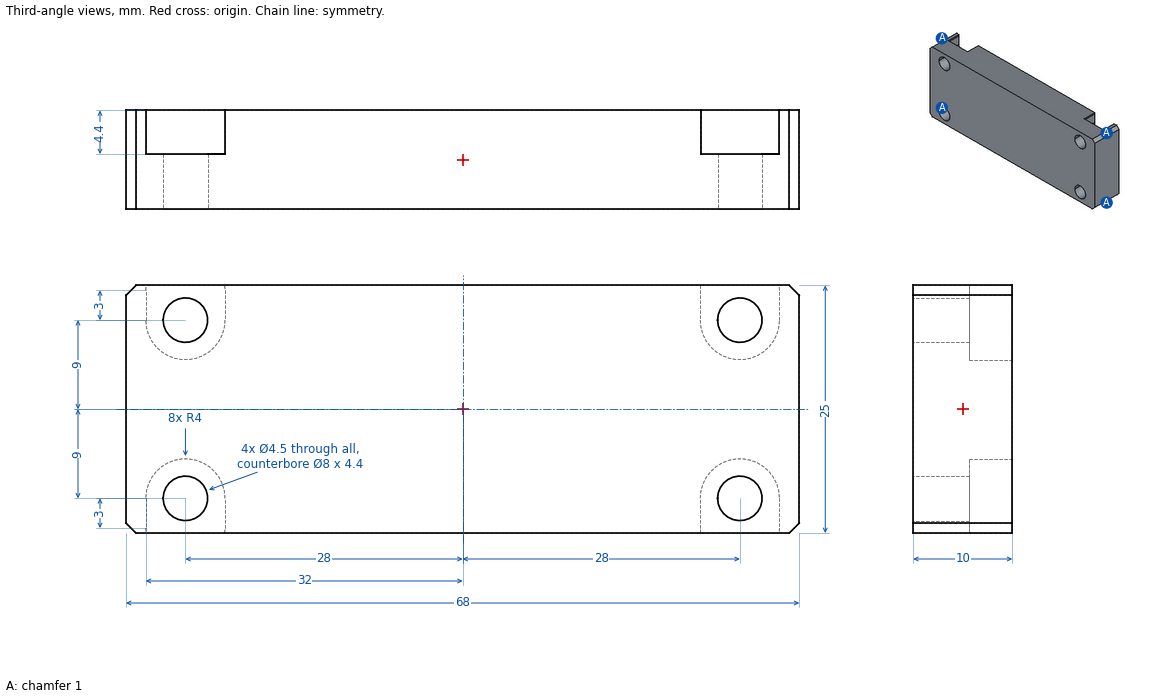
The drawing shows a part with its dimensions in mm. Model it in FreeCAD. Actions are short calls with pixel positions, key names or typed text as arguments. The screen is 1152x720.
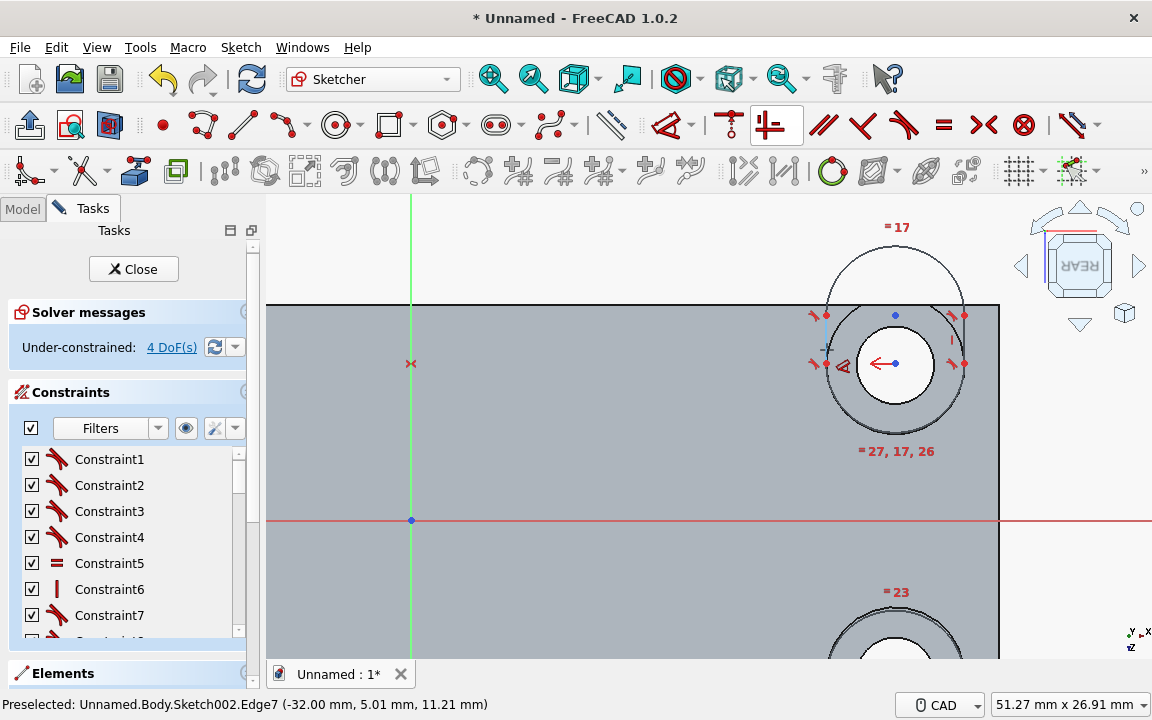
click(826, 349)
click(860, 340)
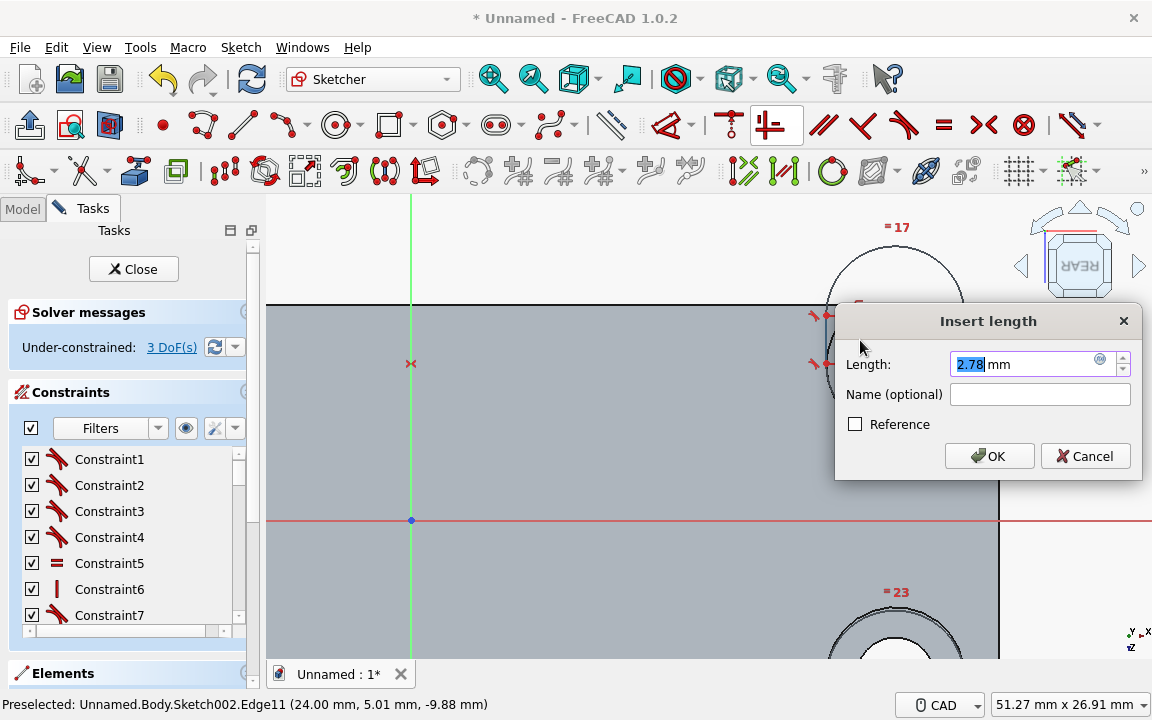
text(3)
key(Return)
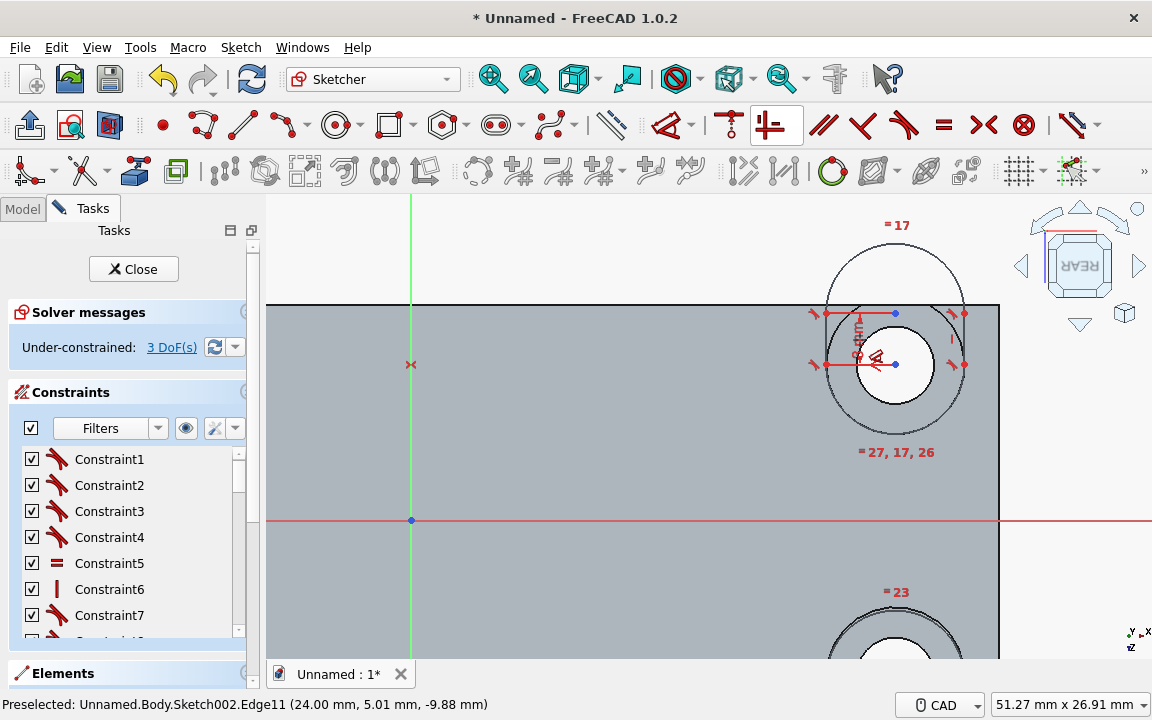
scroll(827, 350, down, 4)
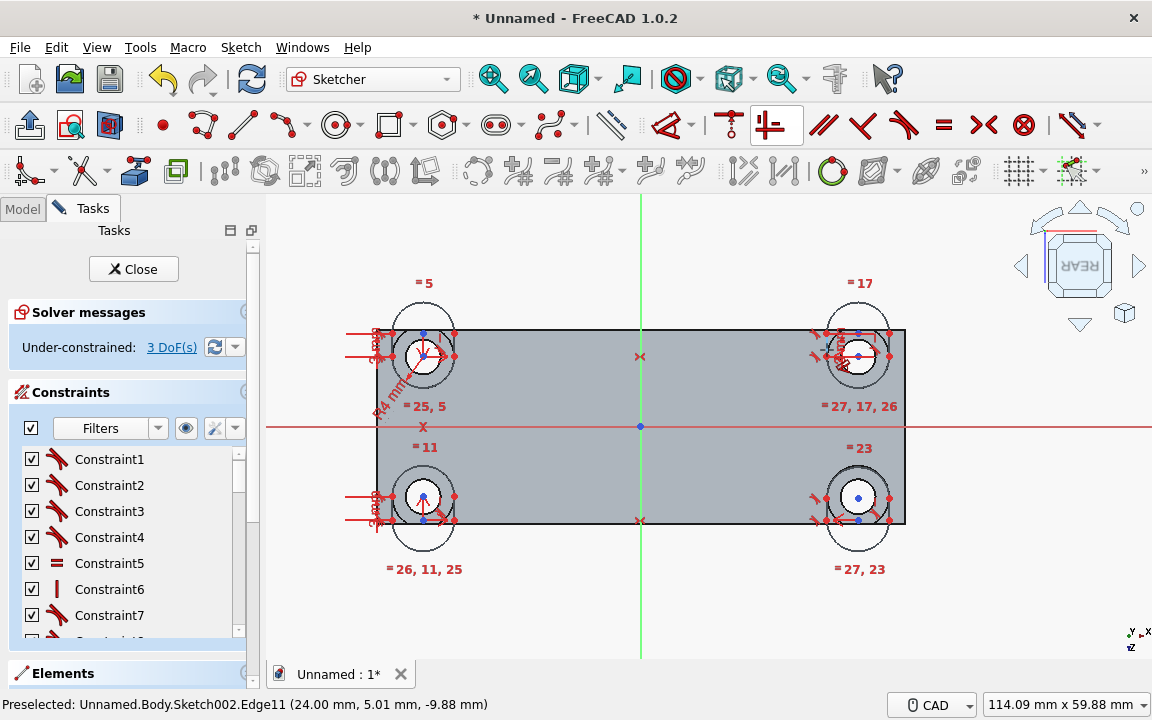
scroll(827, 514, up, 4)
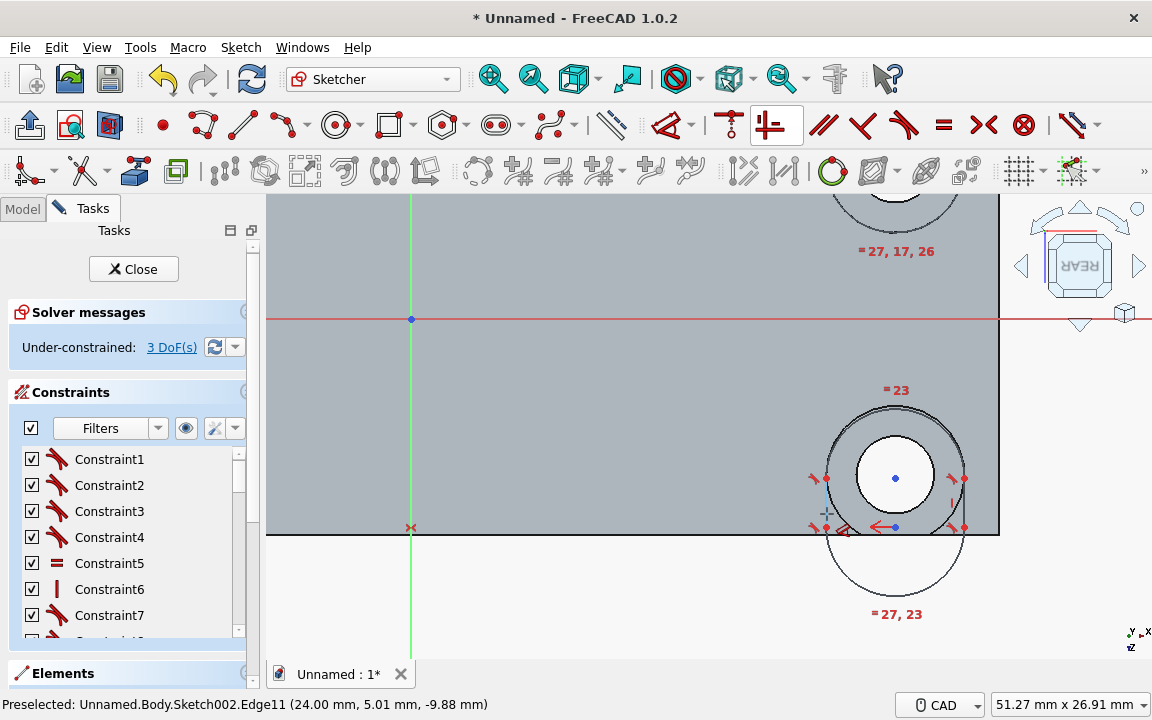
click(826, 512)
click(860, 503)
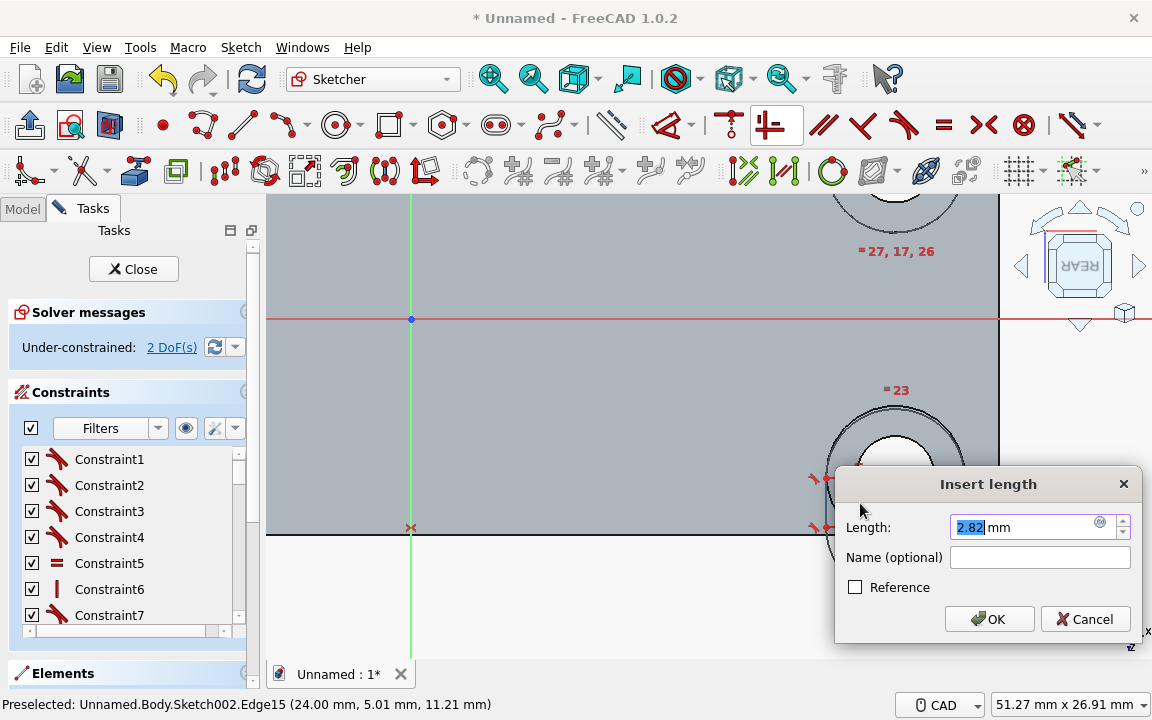
text(3)
key(Return)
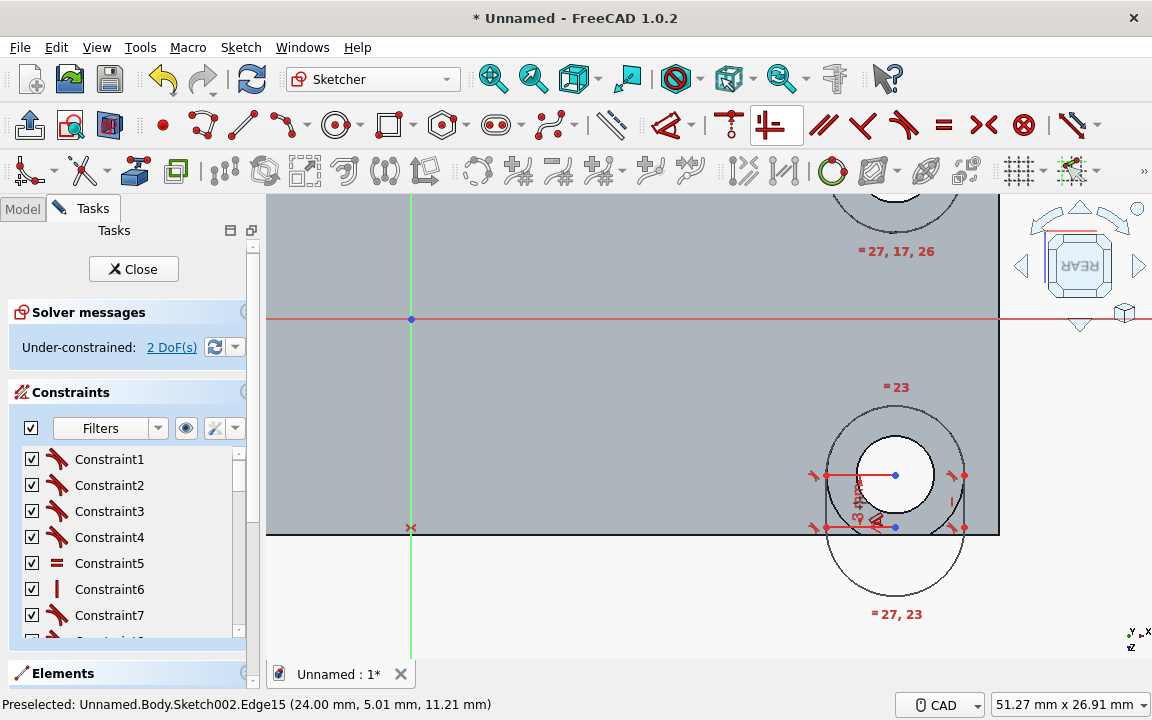
scroll(827, 514, down, 4)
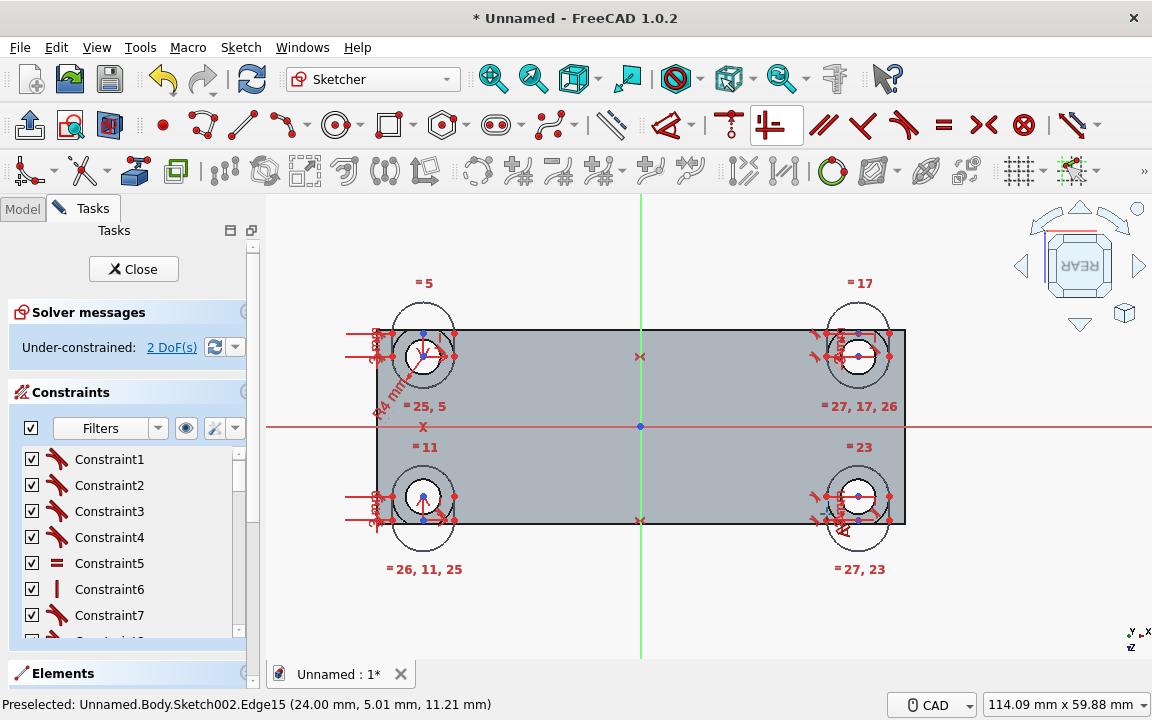
click(392, 357)
click(358, 376)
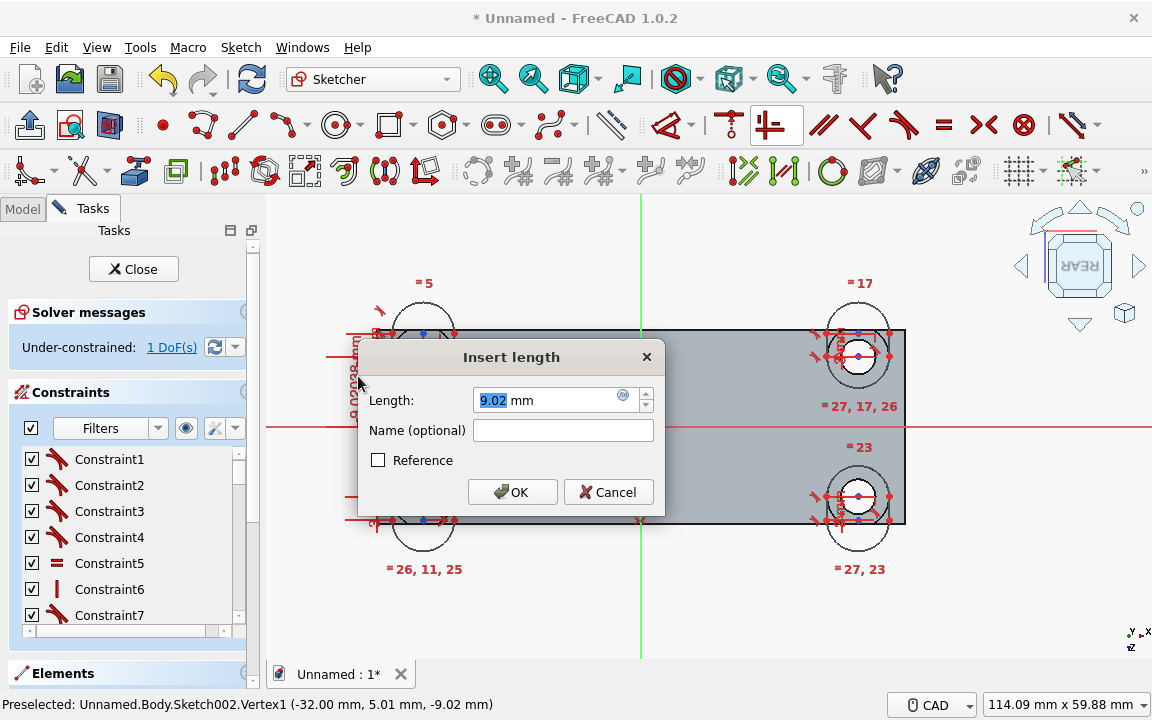
text(9)
key(Return)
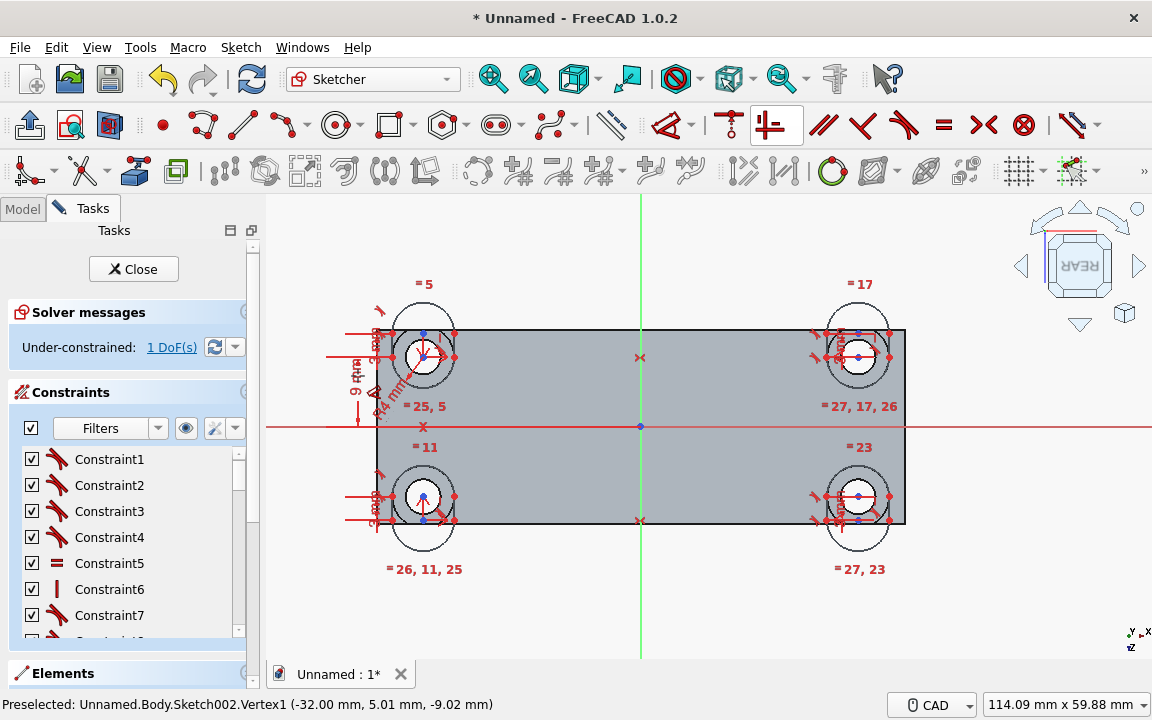
click(392, 357)
click(516, 323)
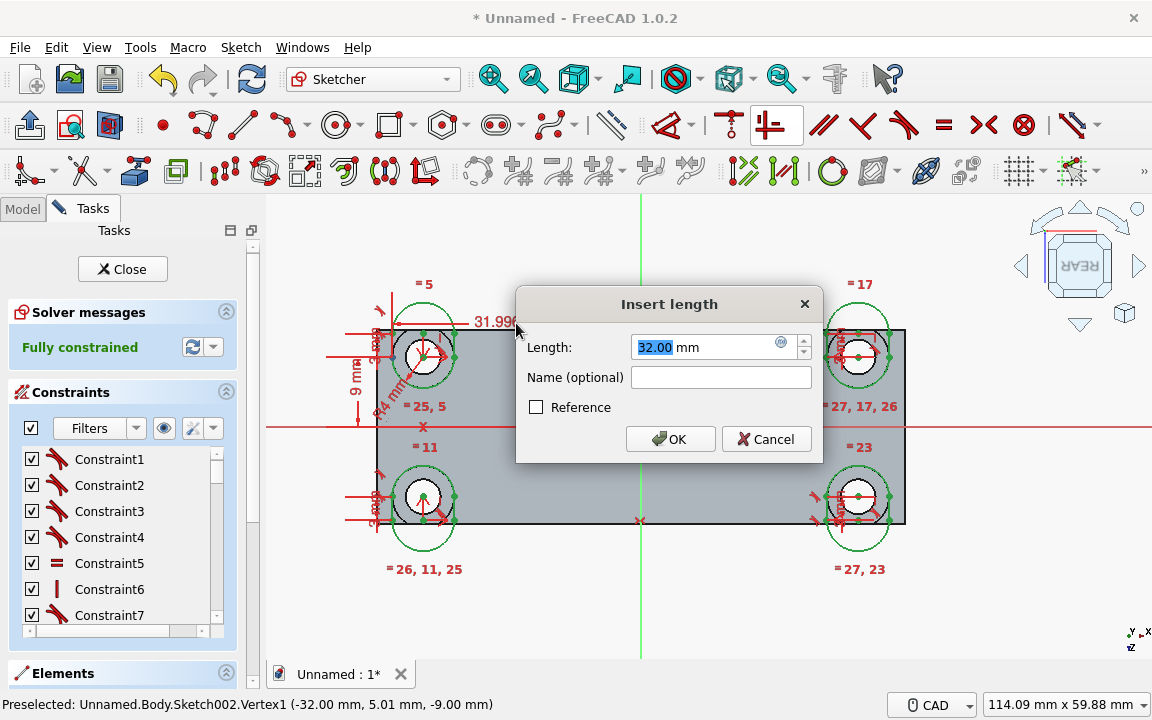
text(32)
key(Return)
key(Escape)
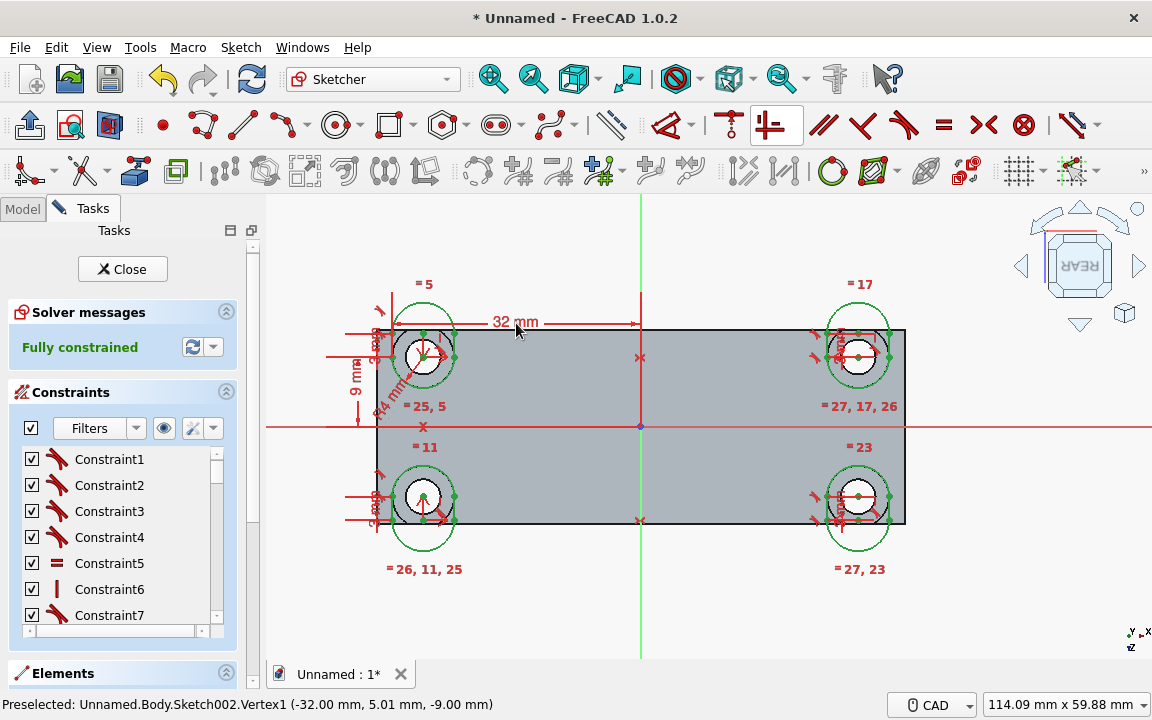
click(123, 269)